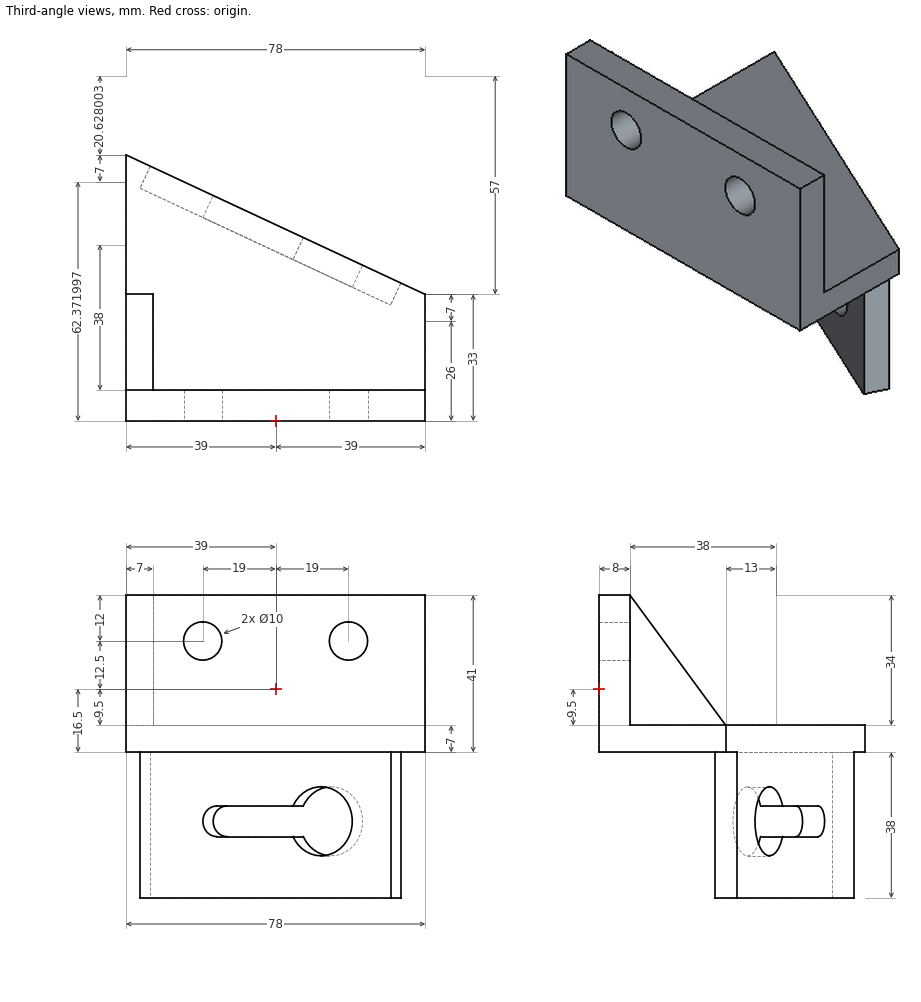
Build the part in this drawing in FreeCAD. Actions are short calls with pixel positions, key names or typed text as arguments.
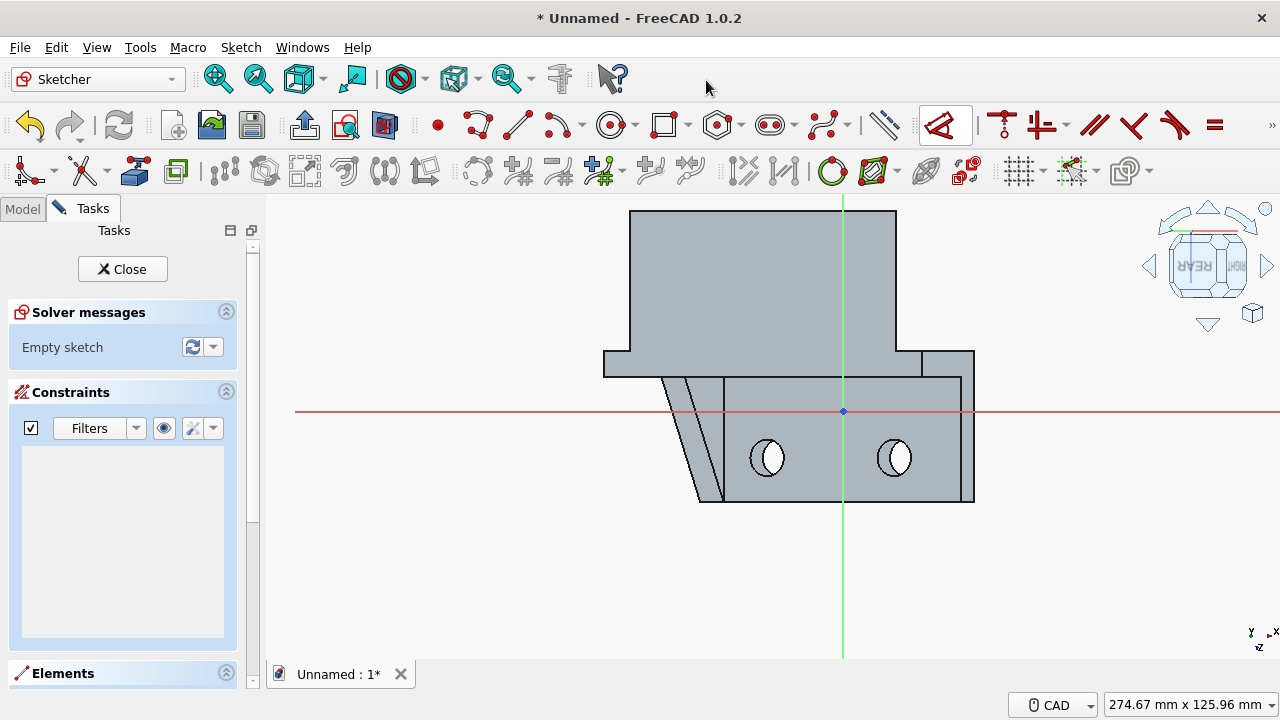
click(386, 126)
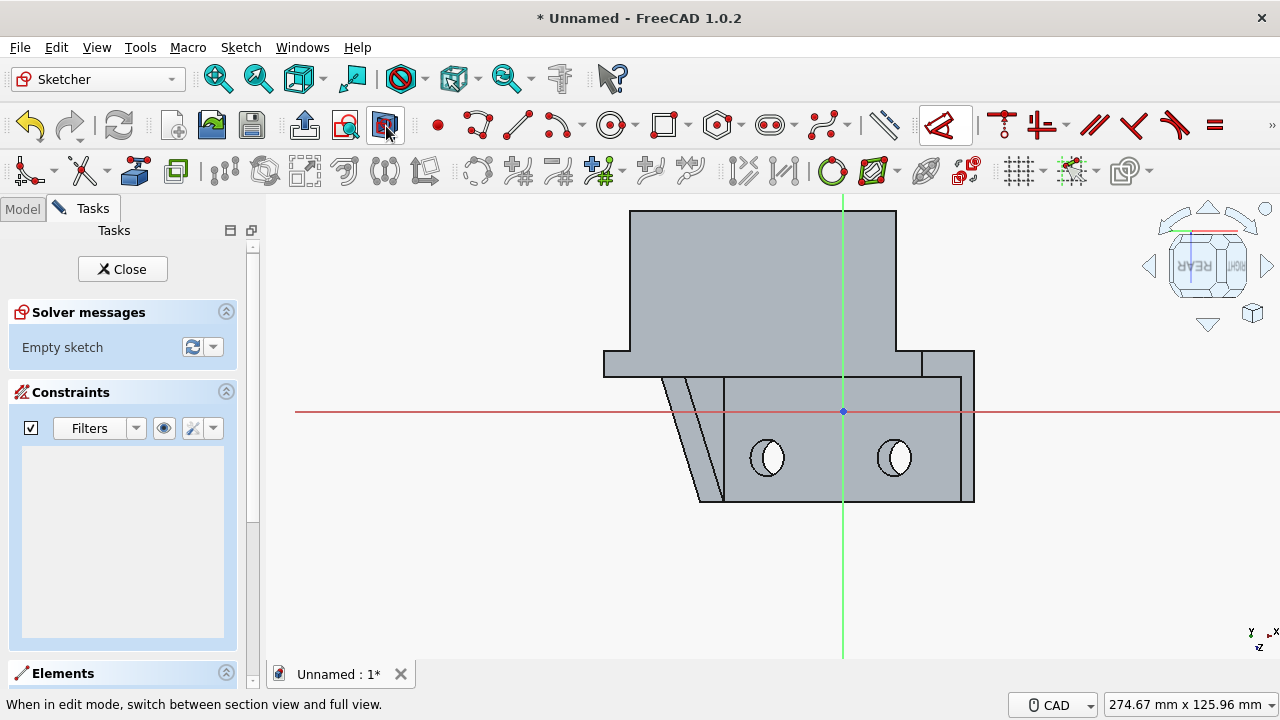
scroll(835, 271, up, 4)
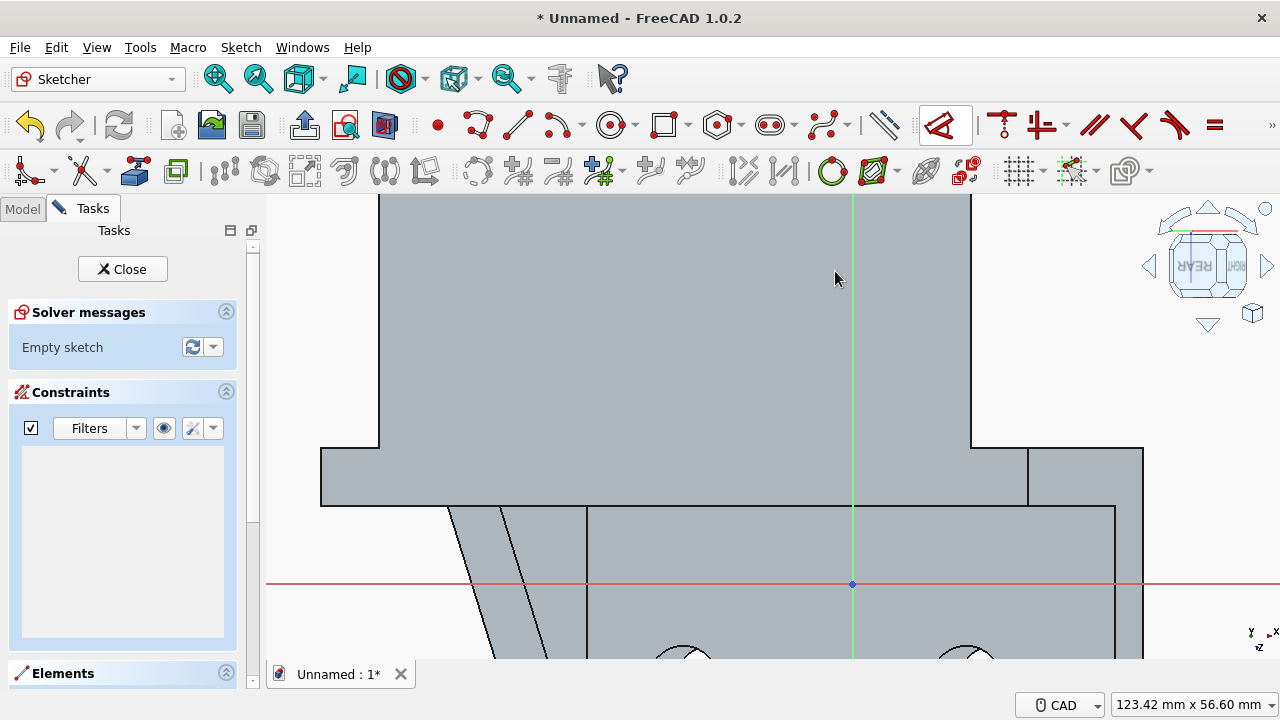
key(g)
key(l)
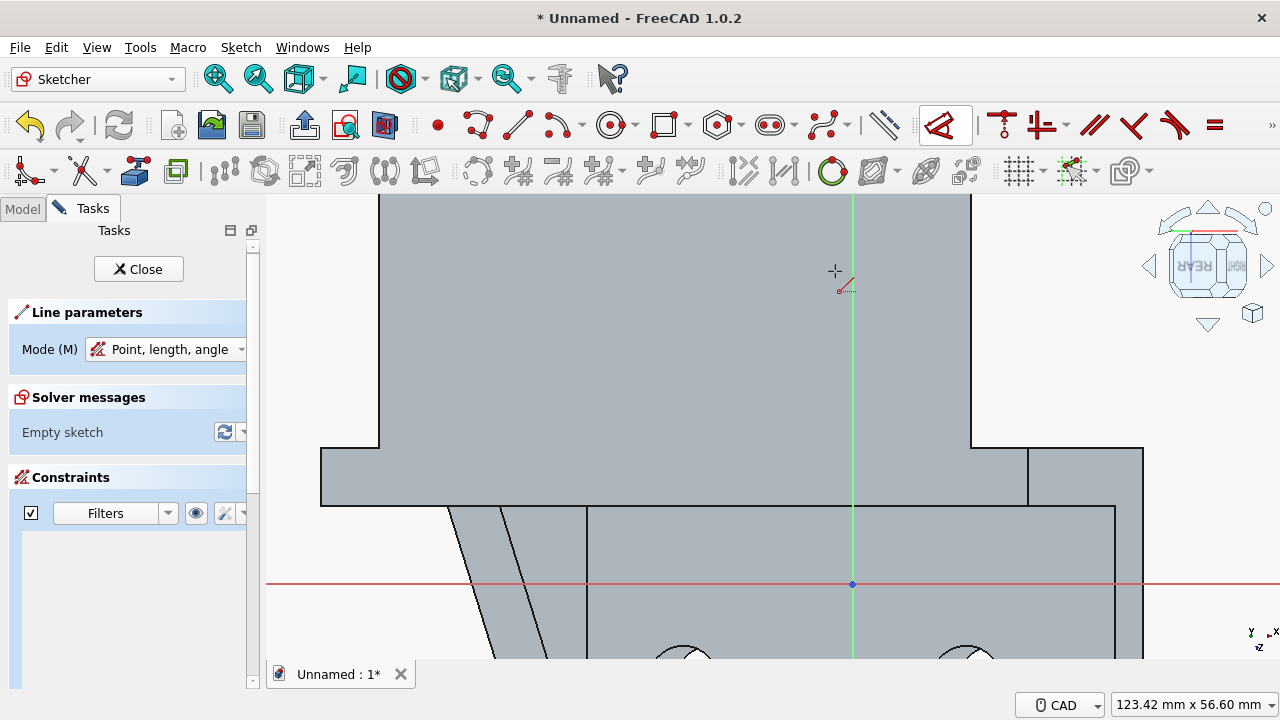
click(740, 268)
click(560, 268)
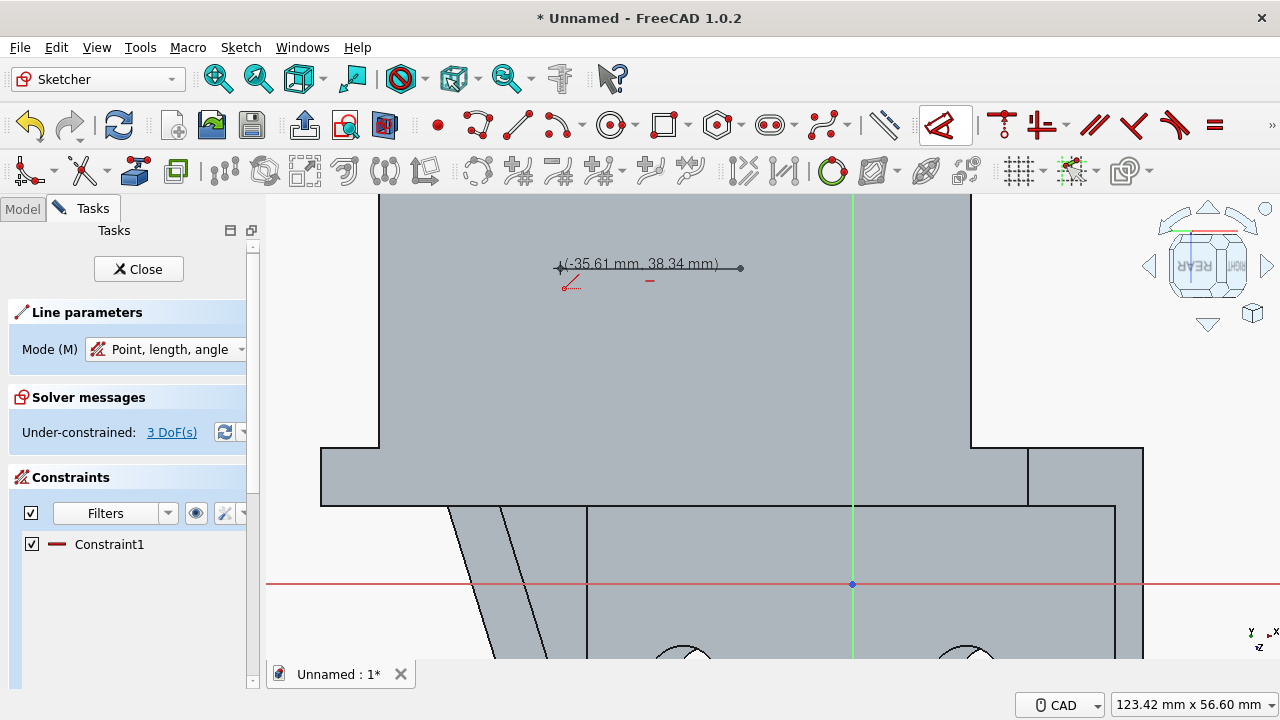
click(560, 333)
click(740, 333)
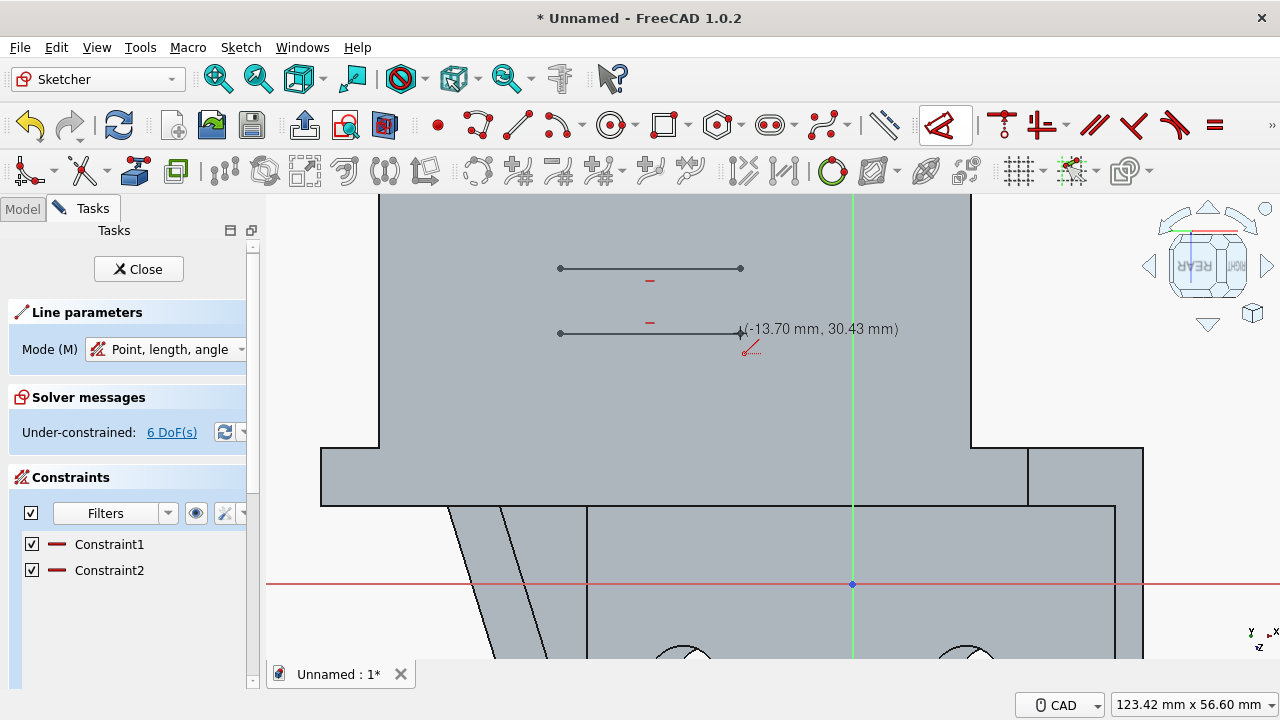
click(584, 126)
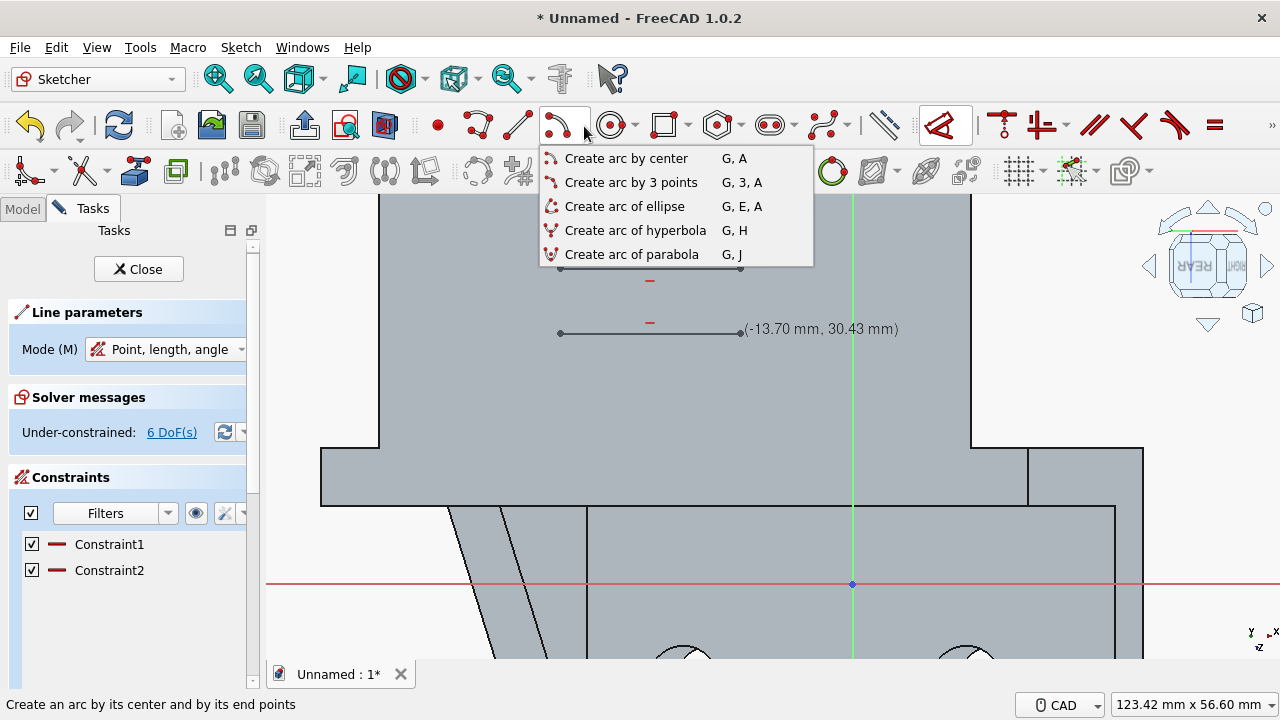
click(676, 182)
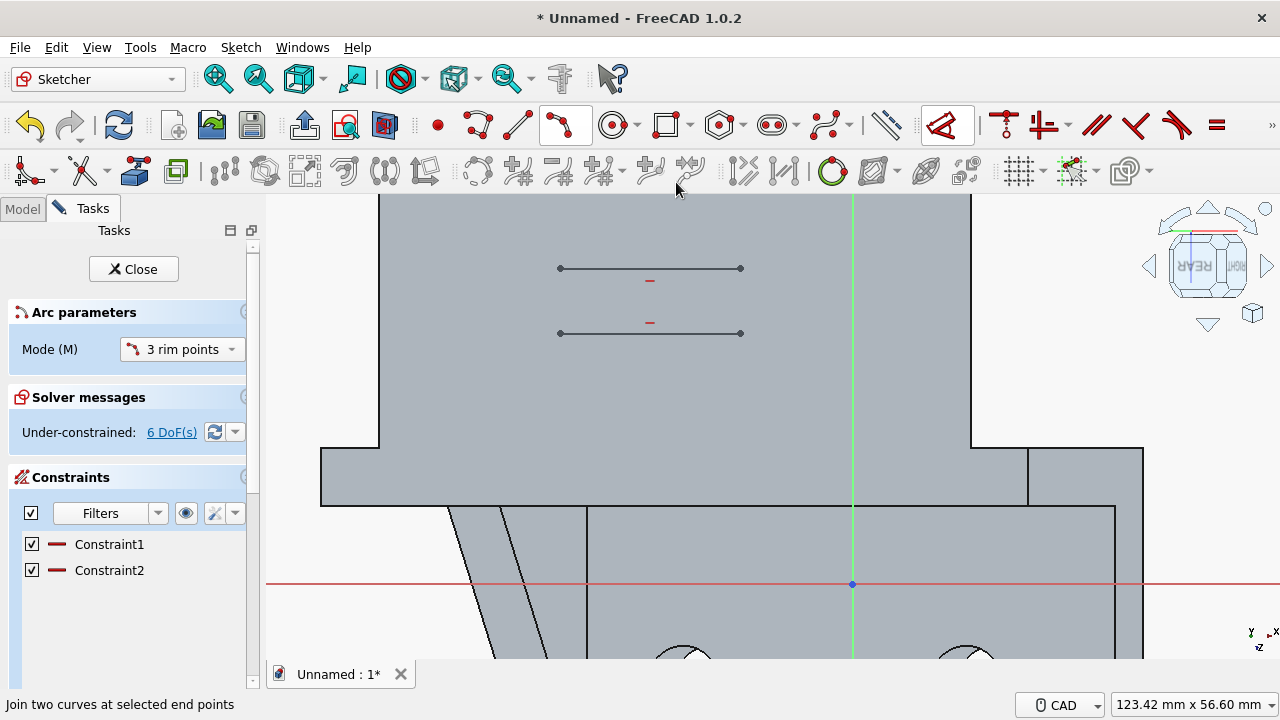
click(560, 269)
click(560, 334)
click(527, 301)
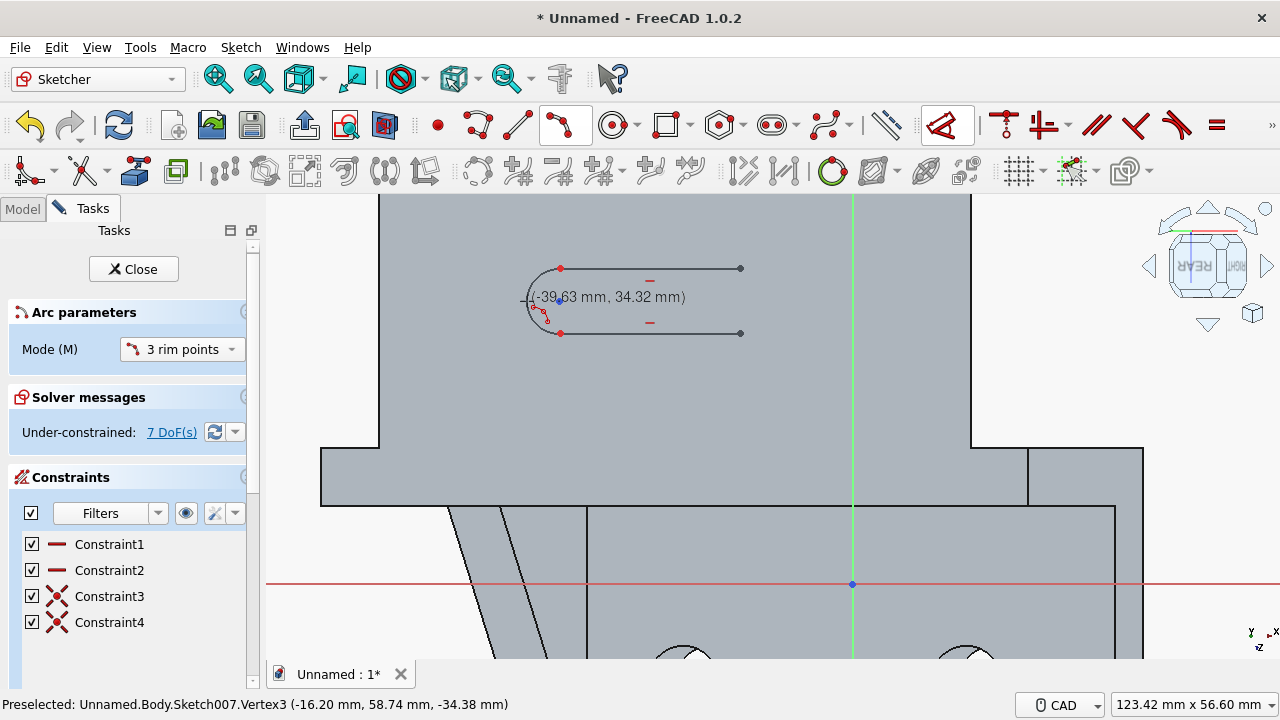
click(740, 334)
click(740, 269)
click(881, 301)
key(Escape)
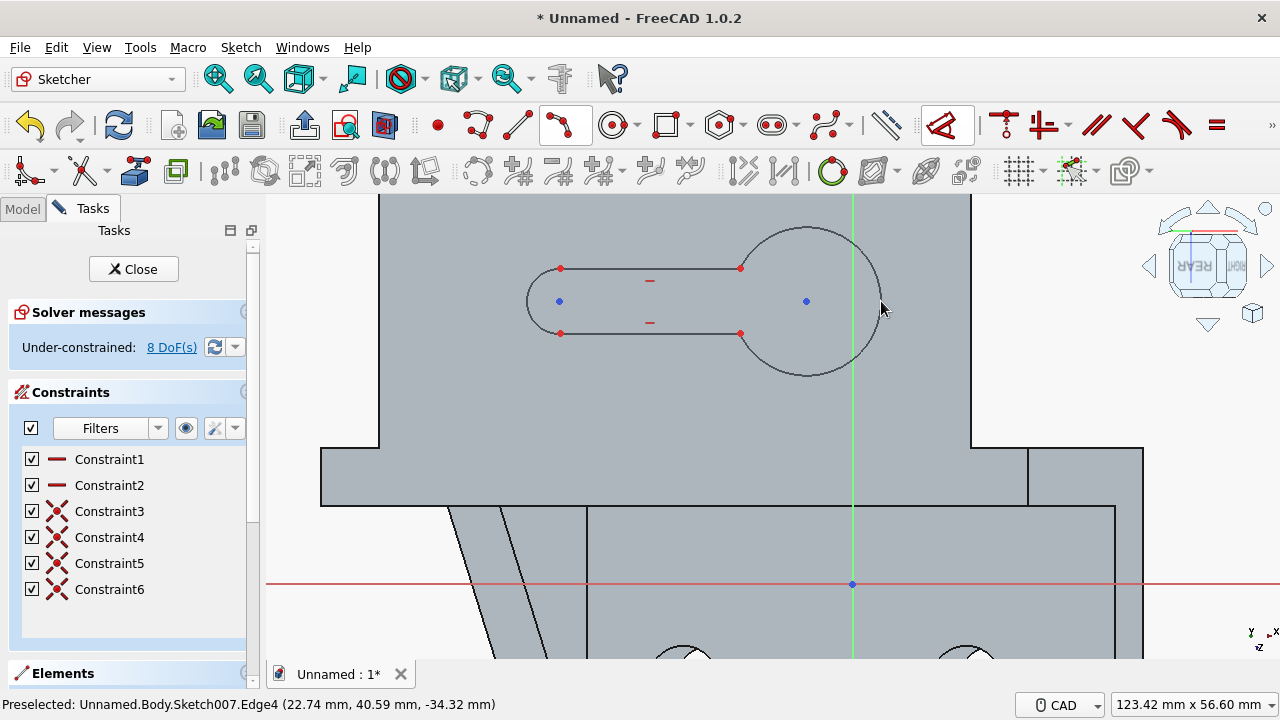
click(686, 269)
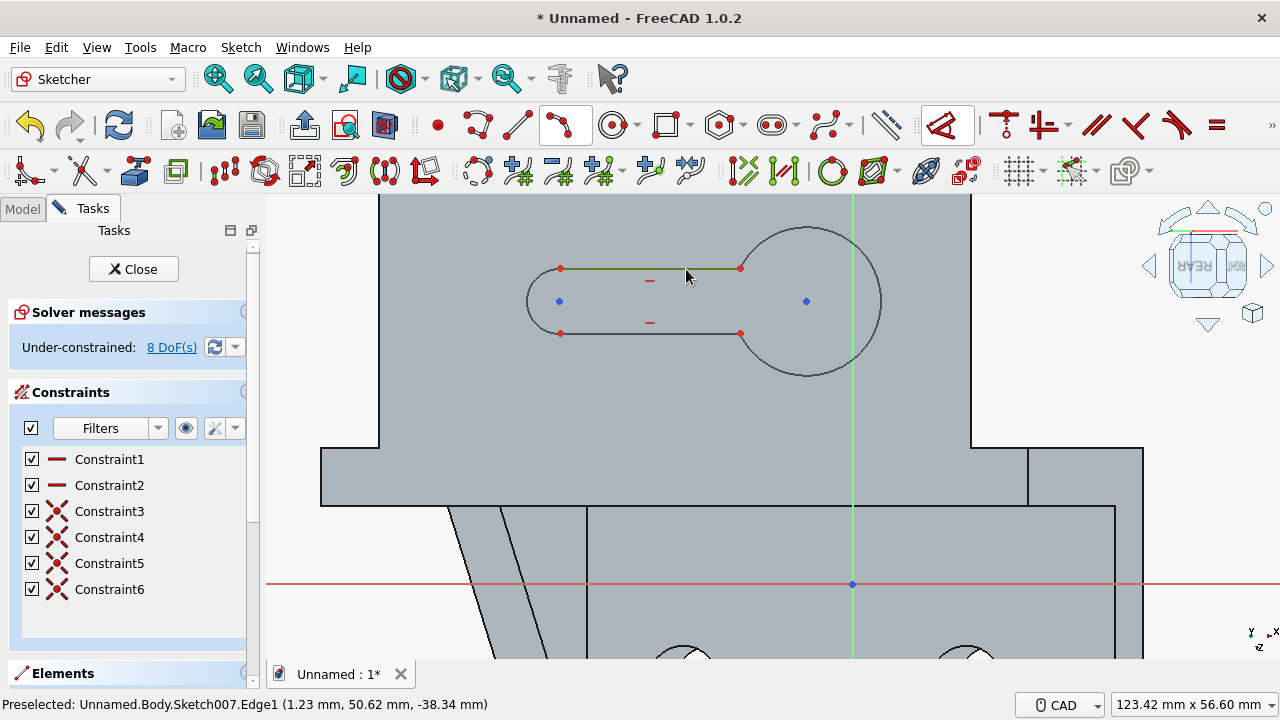
click(533, 282)